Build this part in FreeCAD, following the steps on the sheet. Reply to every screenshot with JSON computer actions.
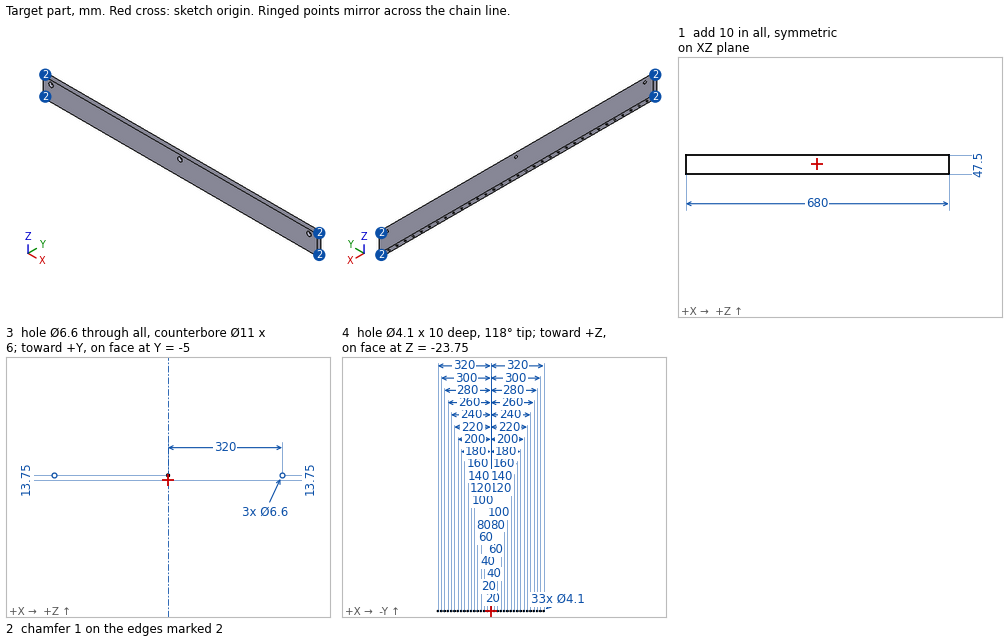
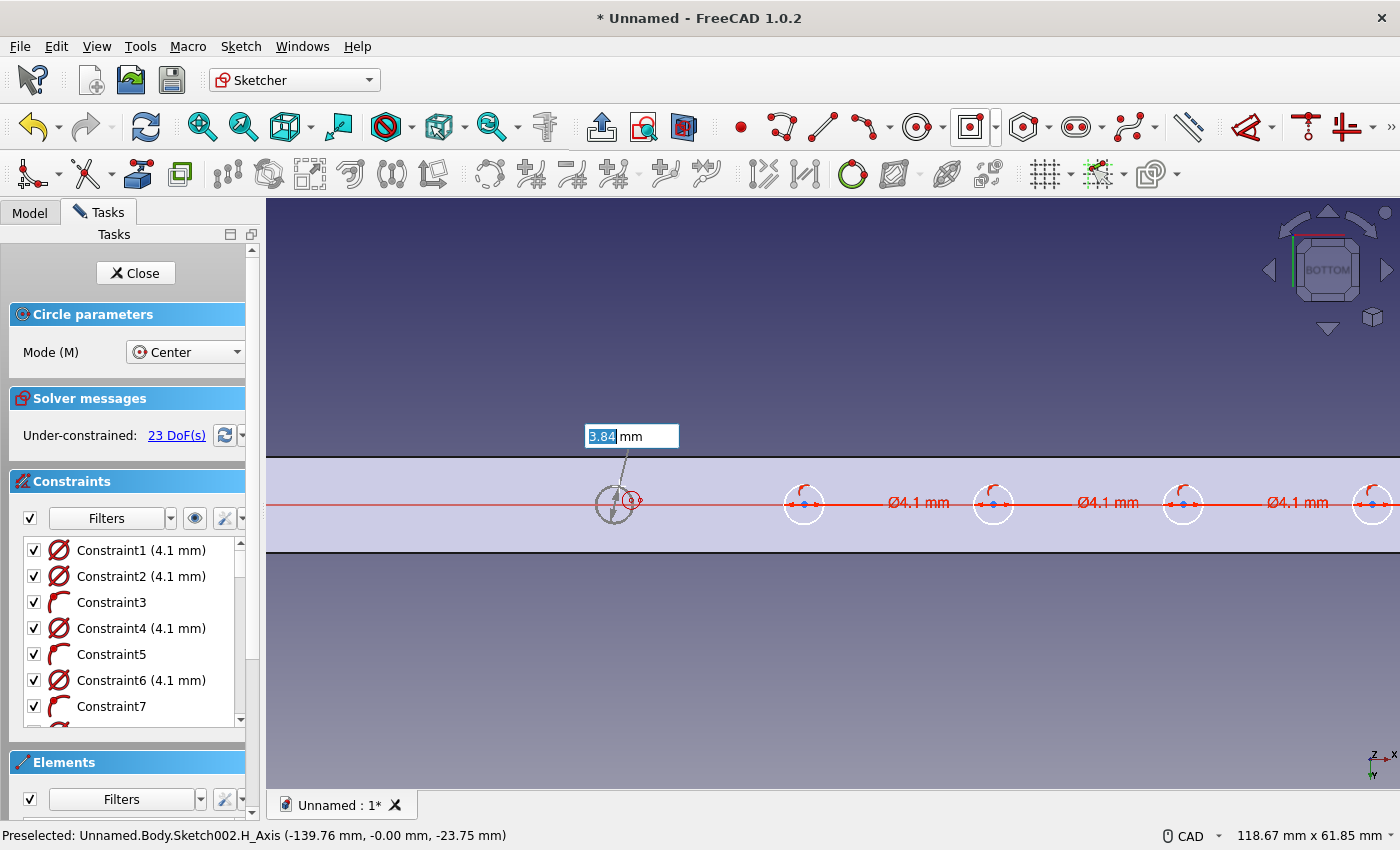
{"action": "type", "text": "4.1"}
{"action": "key", "text": "Return"}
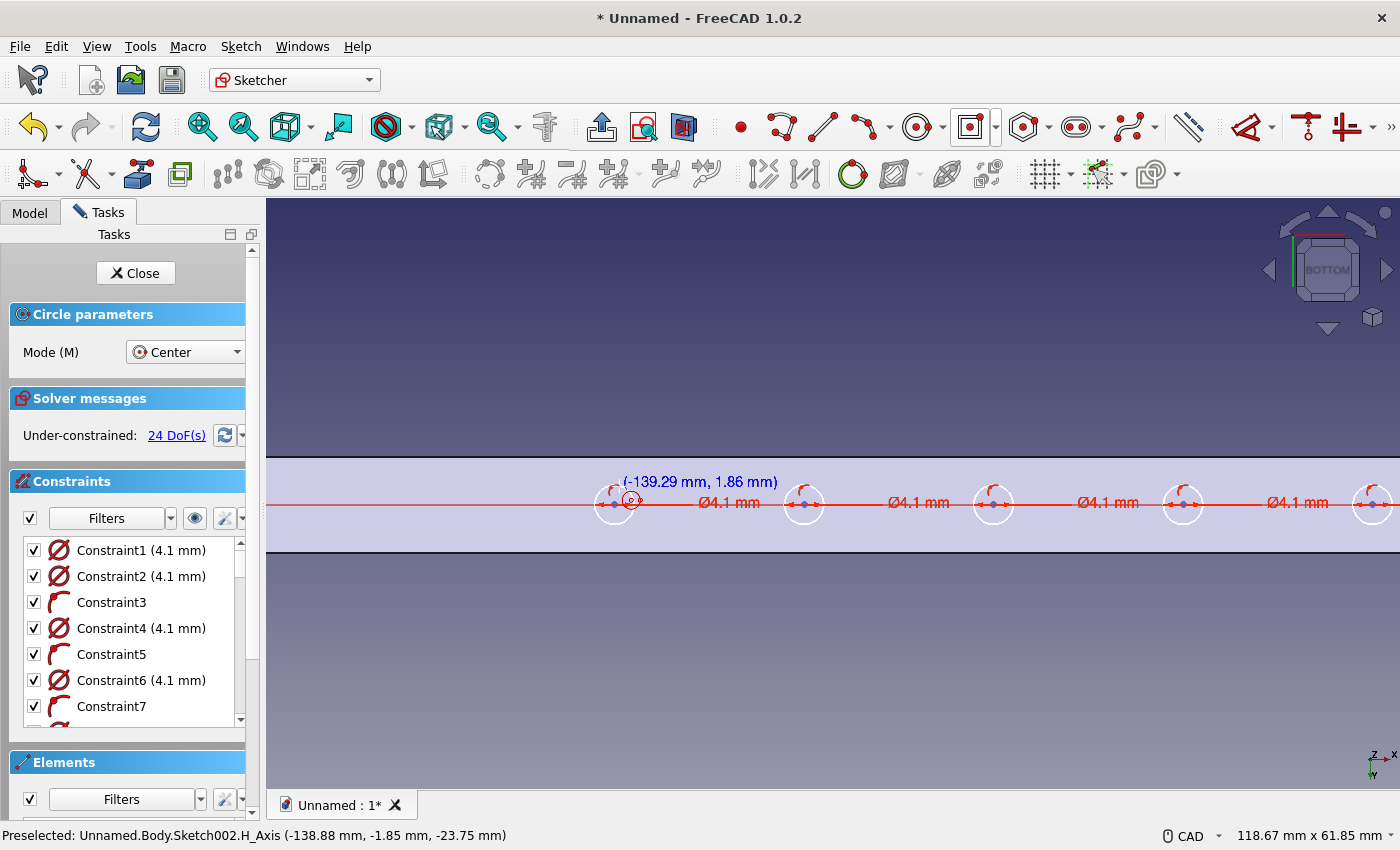
{"action": "scroll", "coordinate": [617, 492], "scroll_direction": "down", "scroll_amount": 11}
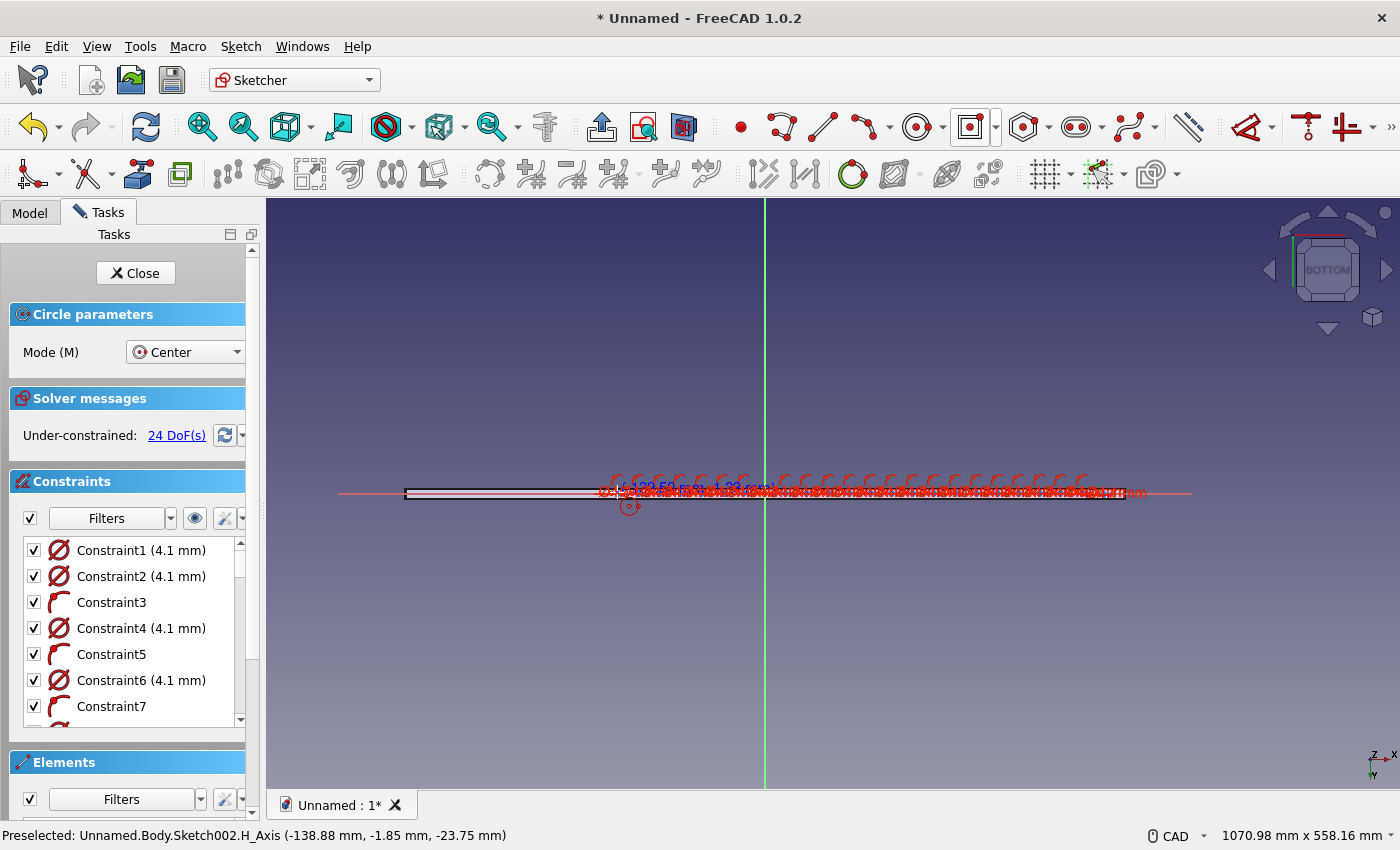
{"action": "left_click", "coordinate": [596, 494]}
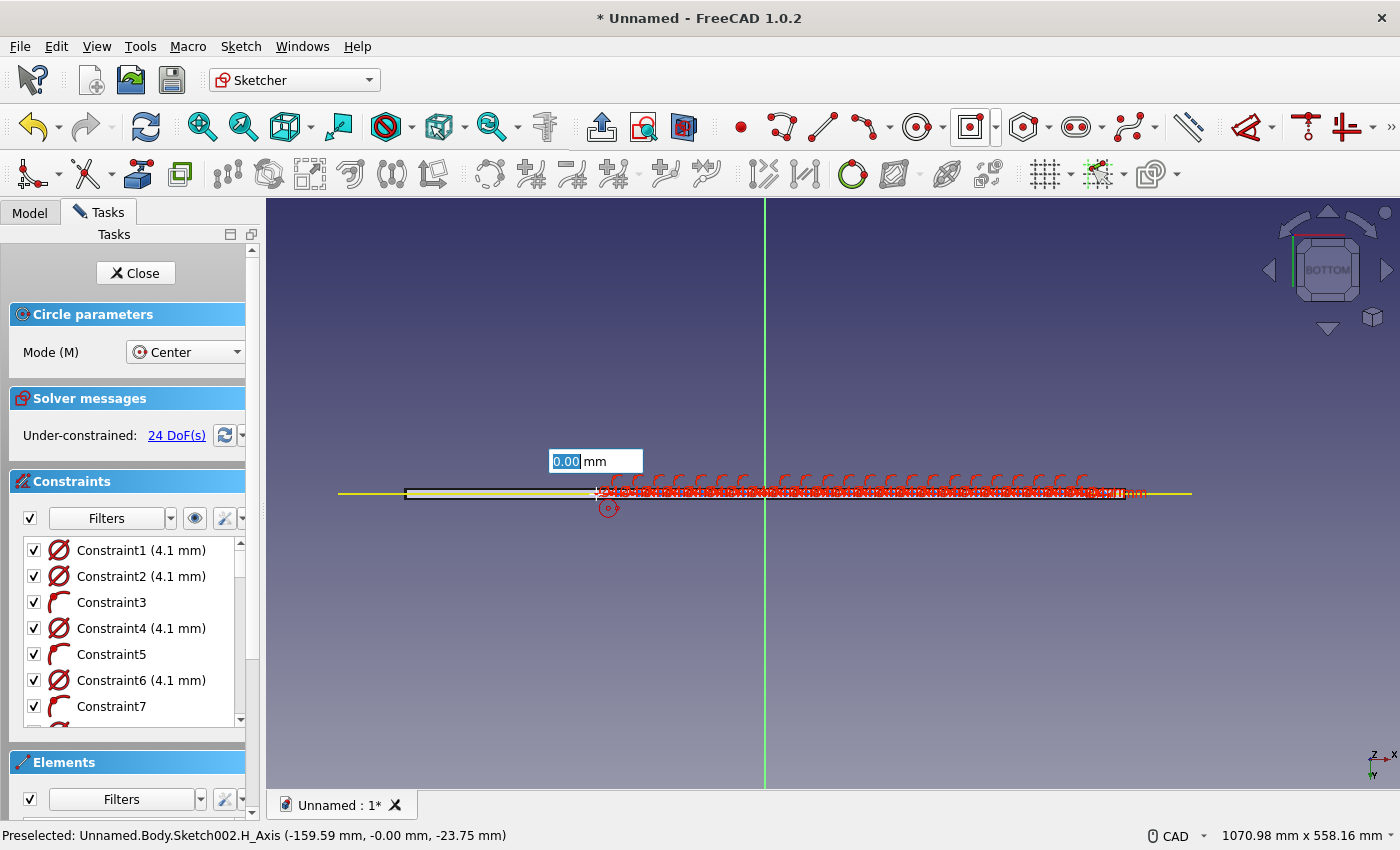
{"action": "scroll", "coordinate": [596, 492], "scroll_direction": "up", "scroll_amount": 11}
{"action": "mouse_move", "coordinate": [596, 486]}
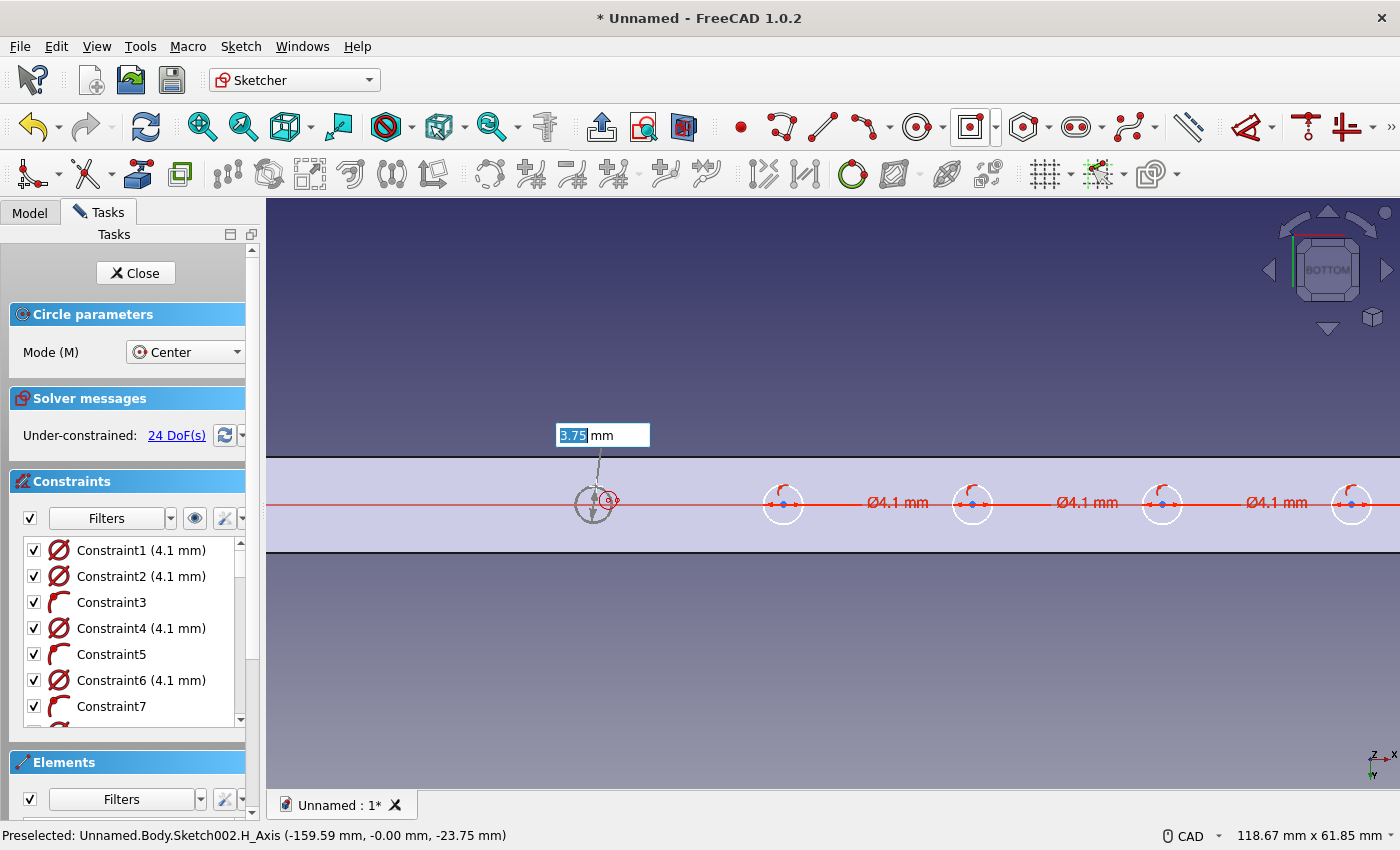
{"action": "type", "text": "4.1"}
{"action": "key", "text": "Return"}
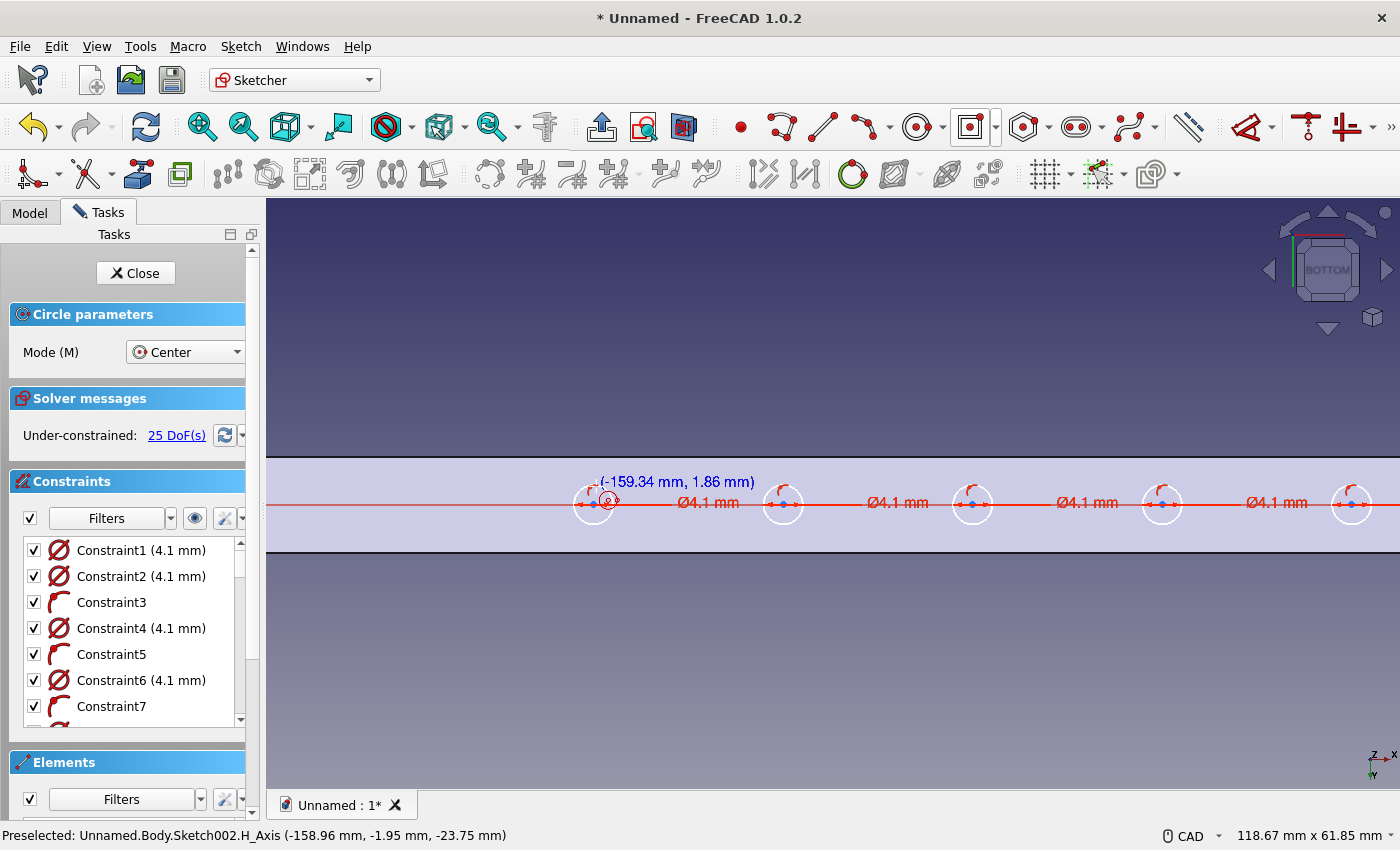
{"action": "scroll", "coordinate": [596, 492], "scroll_direction": "down", "scroll_amount": 11}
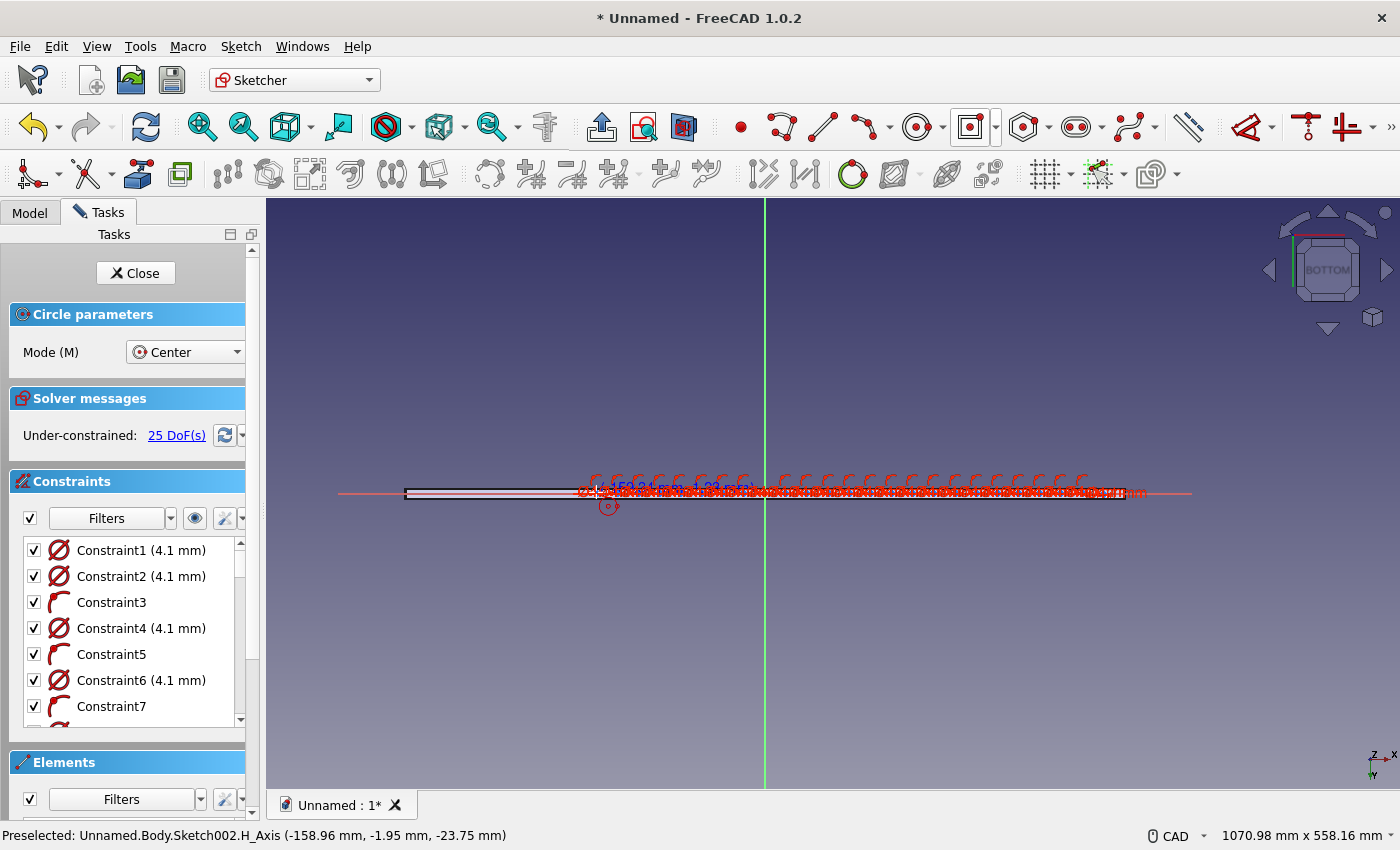
{"action": "left_click", "coordinate": [574, 494]}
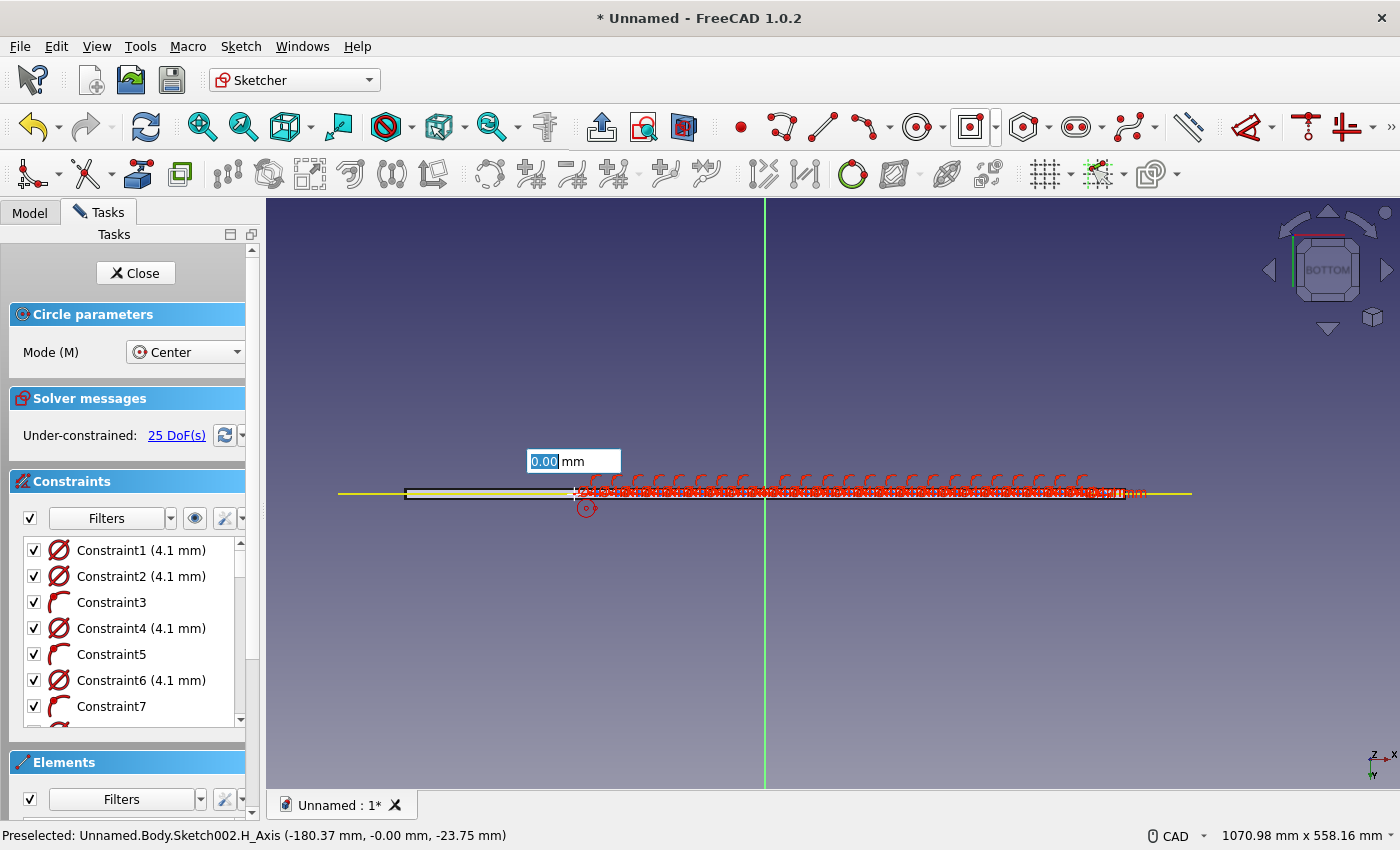
{"action": "scroll", "coordinate": [575, 492], "scroll_direction": "up", "scroll_amount": 11}
{"action": "mouse_move", "coordinate": [574, 486]}